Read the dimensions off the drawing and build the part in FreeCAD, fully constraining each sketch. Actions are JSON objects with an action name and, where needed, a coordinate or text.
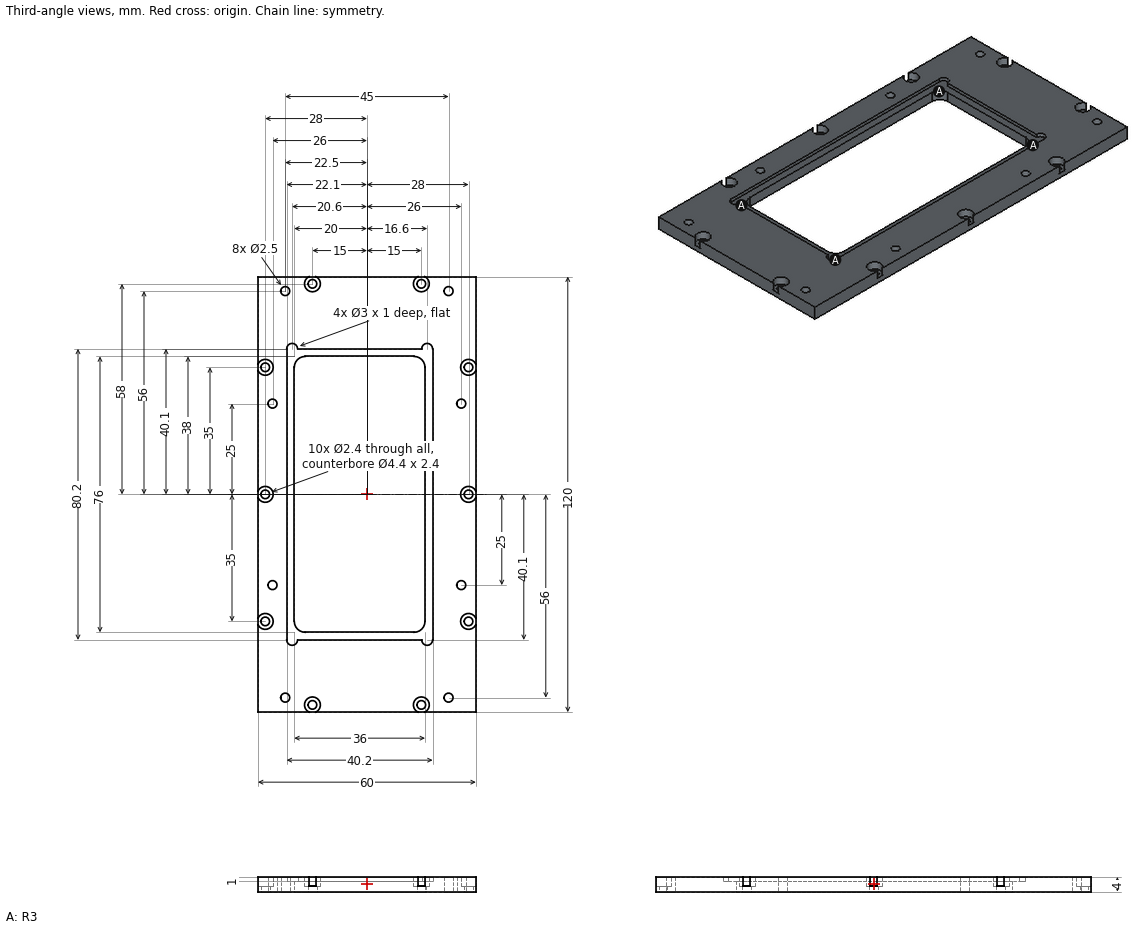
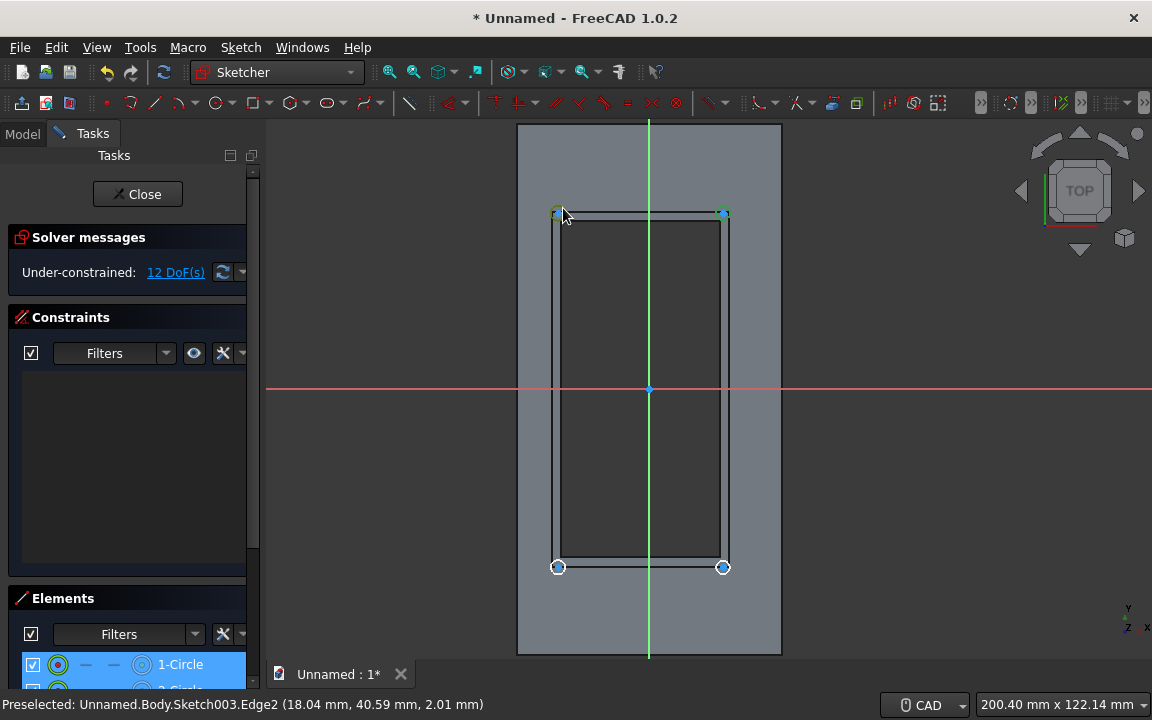
{"action": "scroll", "coordinate": [728, 563], "scroll_direction": "up", "scroll_amount": 4}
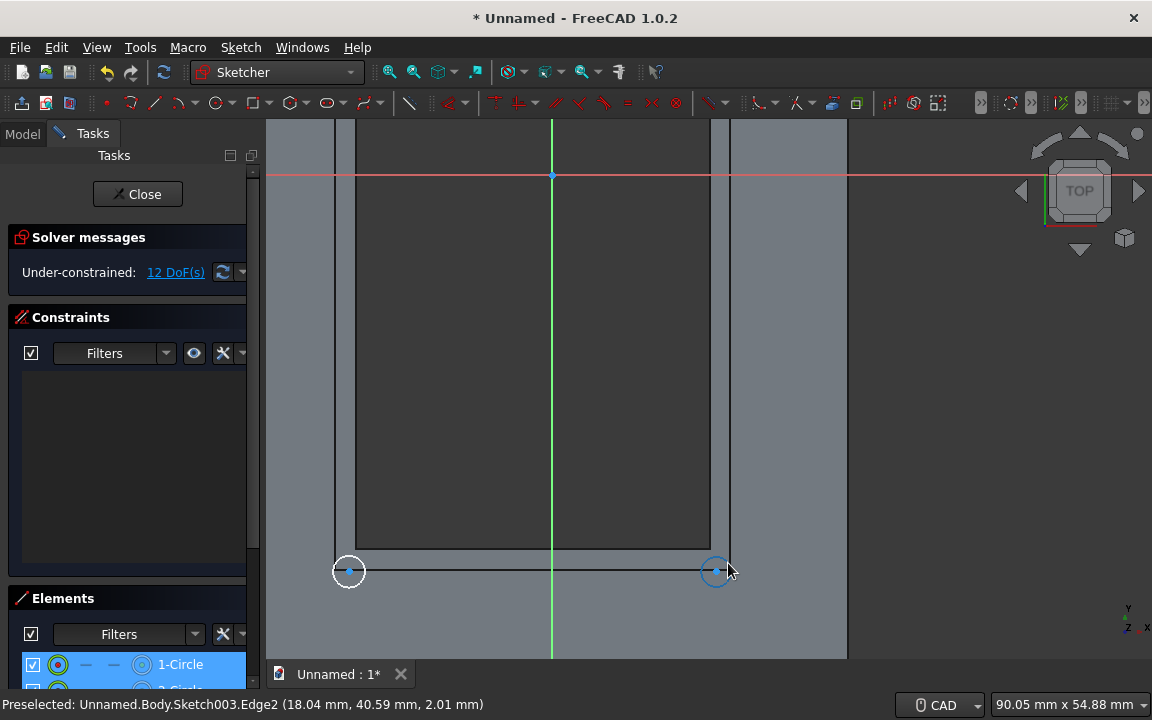
{"action": "left_click", "coordinate": [727, 561]}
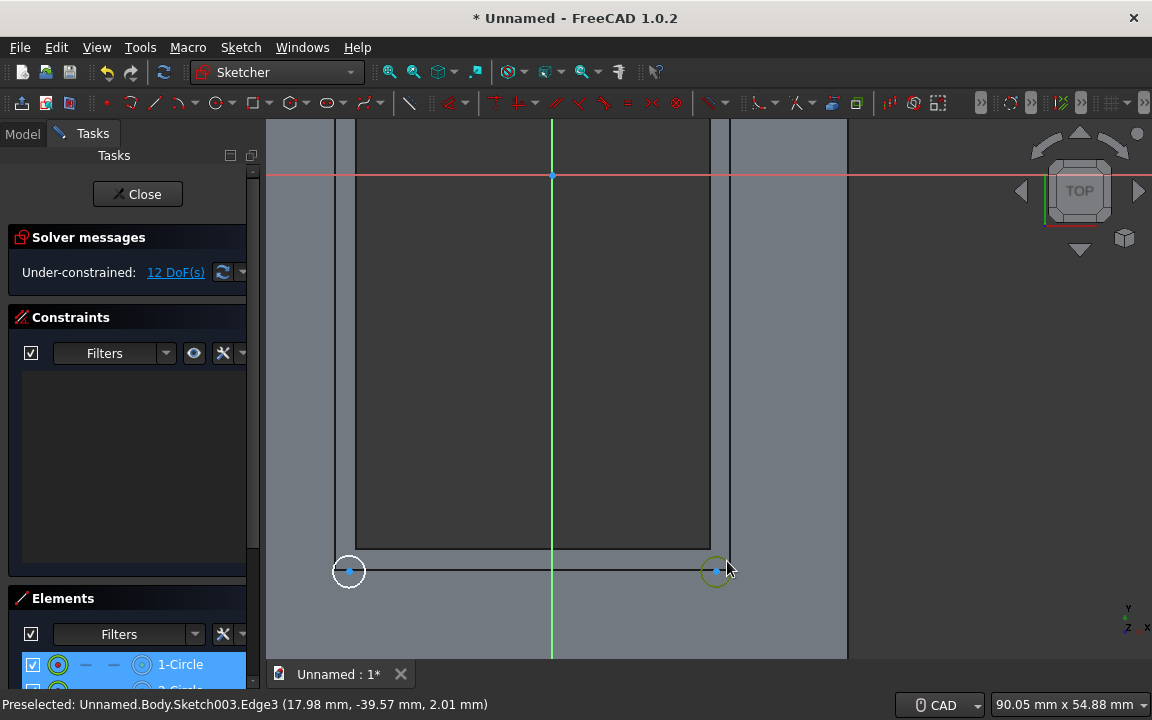
{"action": "left_click", "coordinate": [360, 560]}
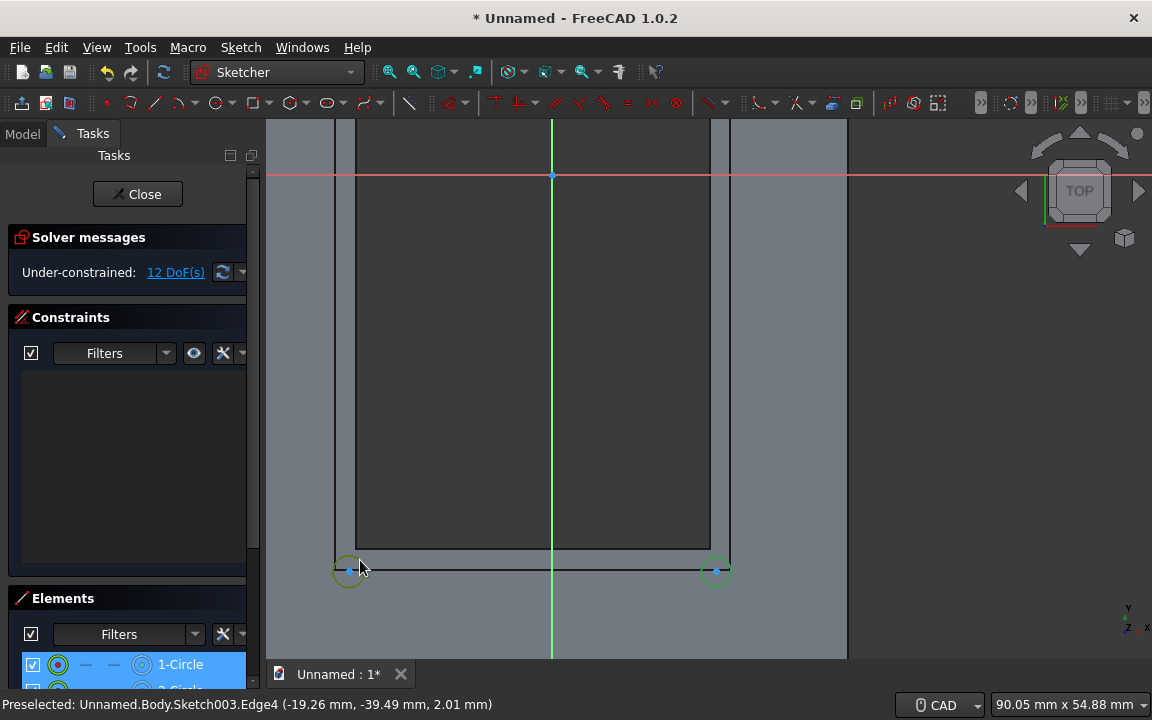
{"action": "key", "text": "e"}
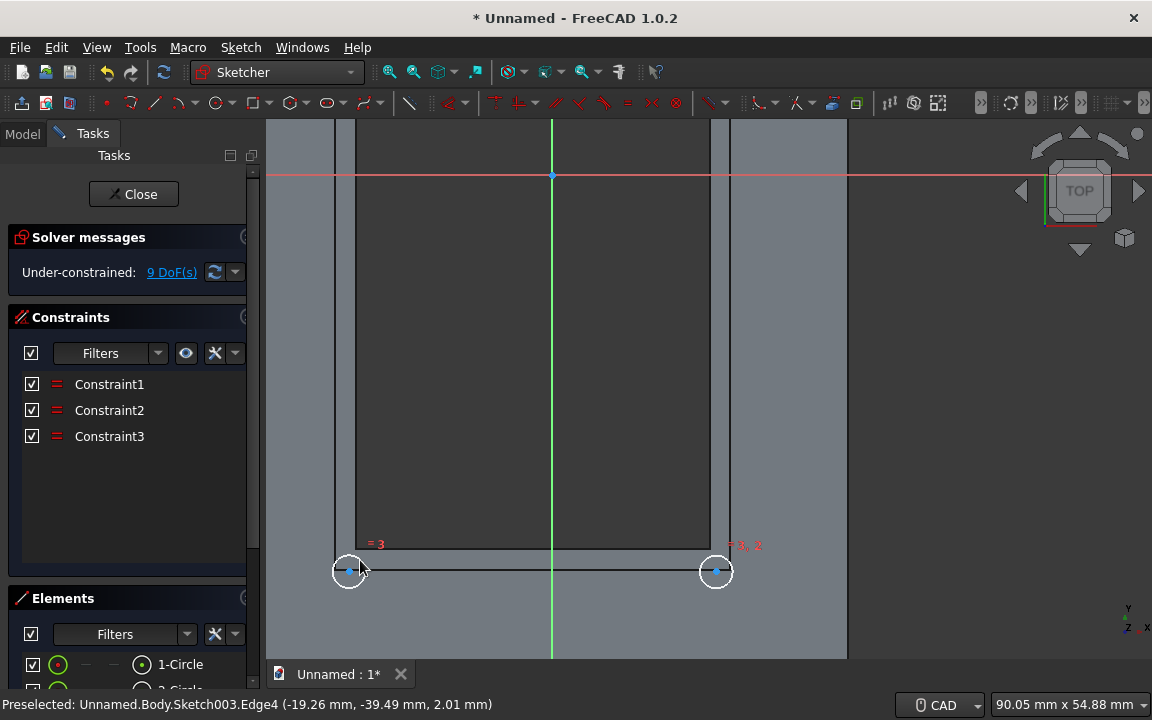
{"action": "scroll", "coordinate": [728, 563], "scroll_direction": "down", "scroll_amount": 4}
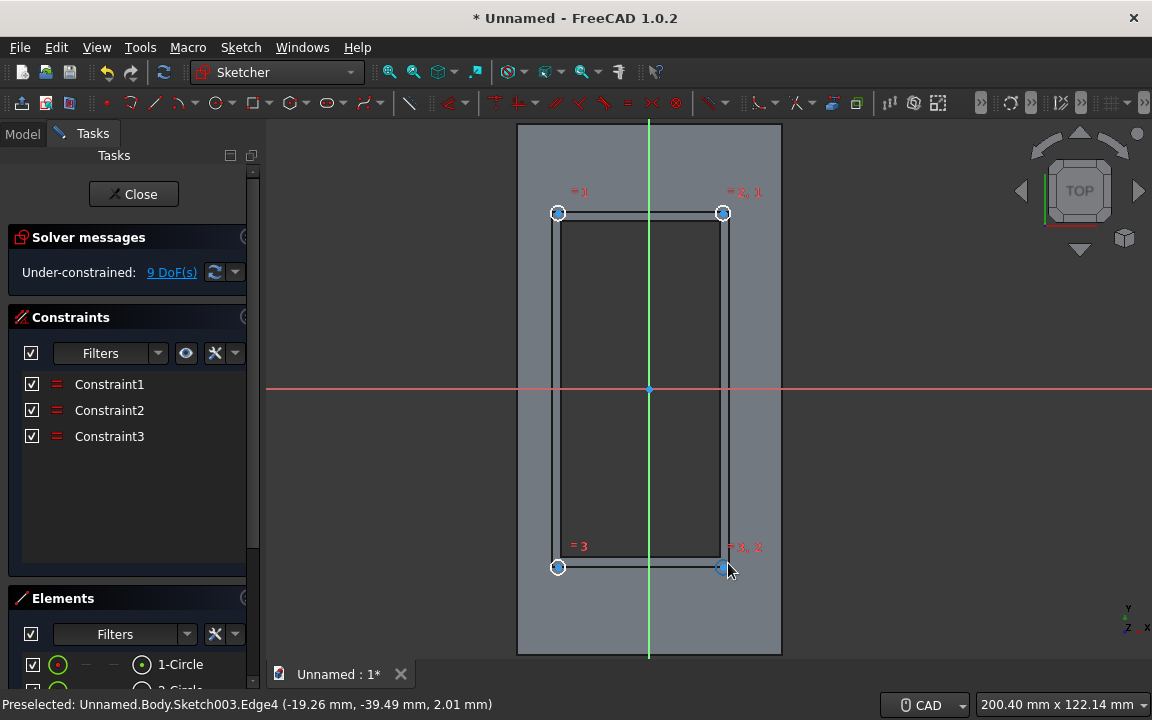
{"action": "left_click", "coordinate": [558, 213]}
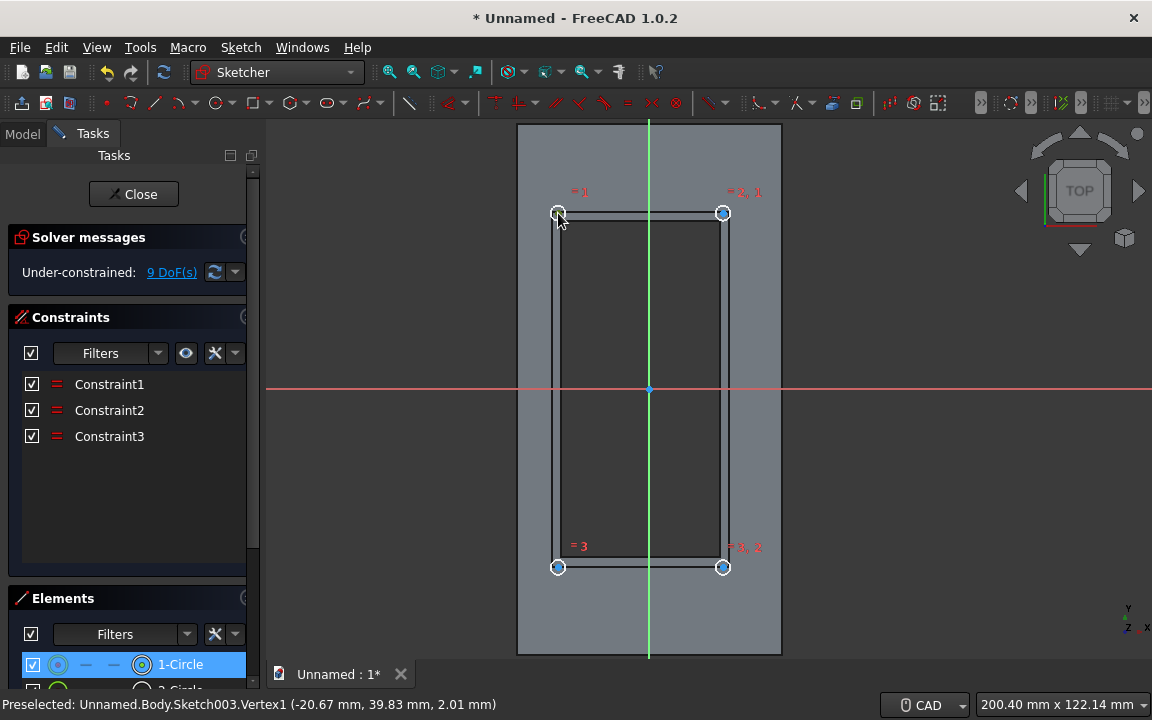
{"action": "left_click", "coordinate": [723, 213]}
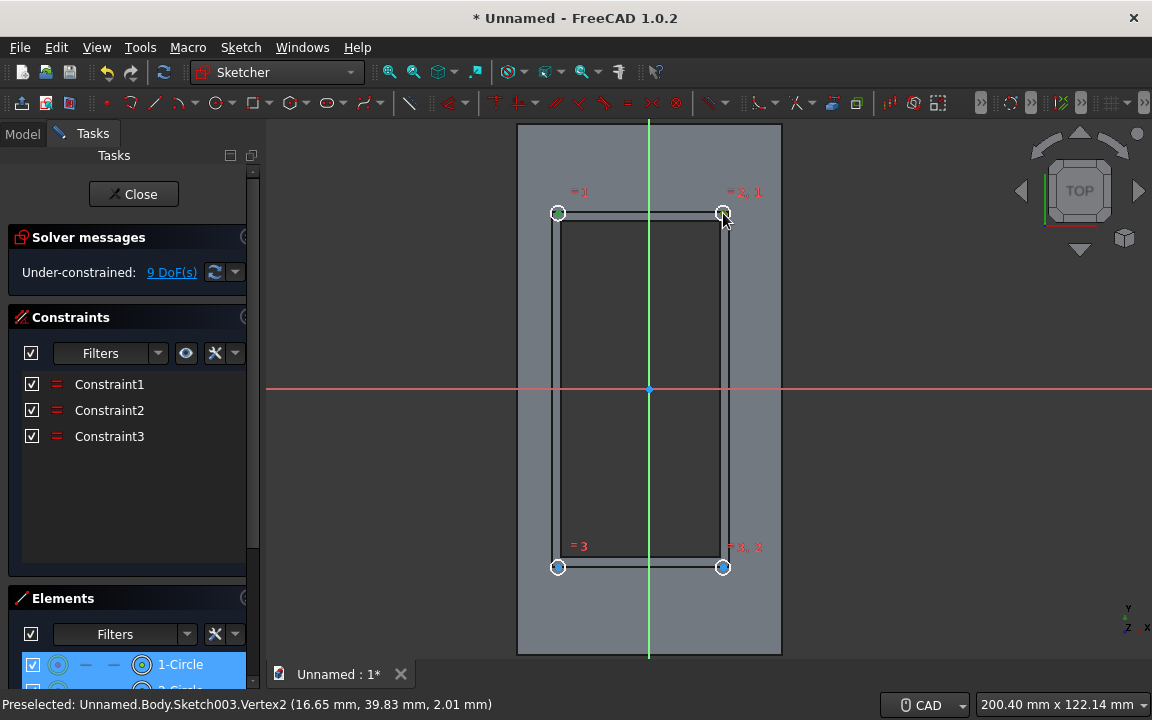
{"action": "key", "text": "h"}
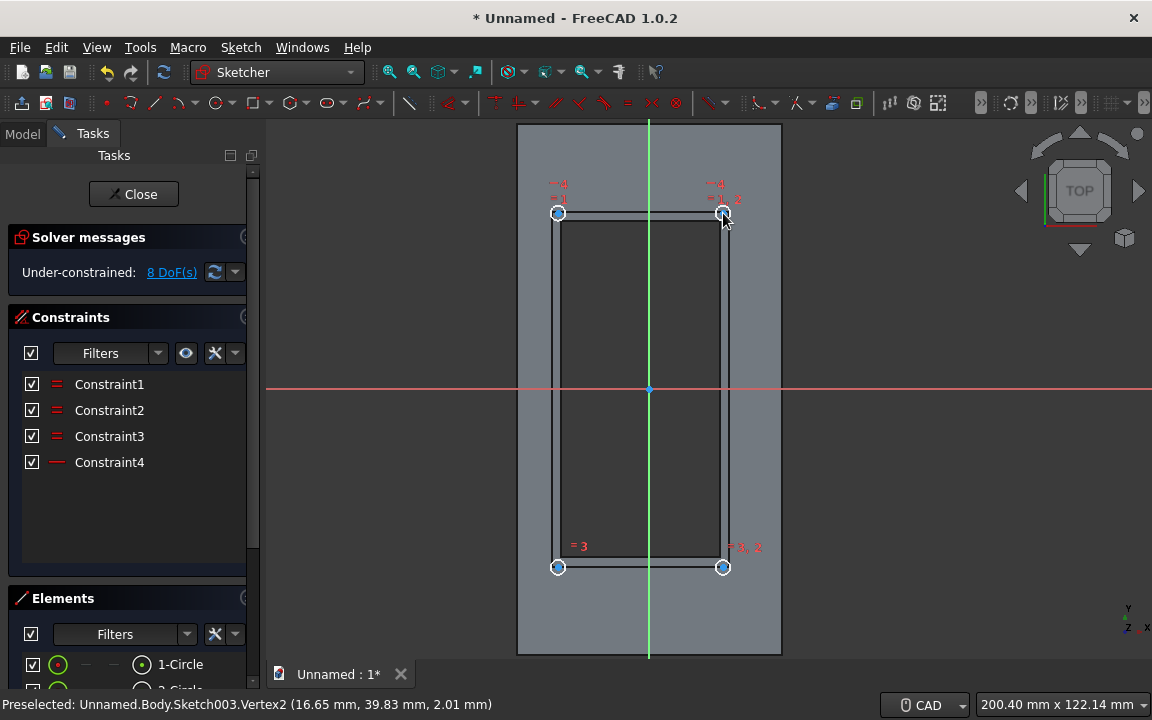
{"action": "left_click", "coordinate": [723, 213]}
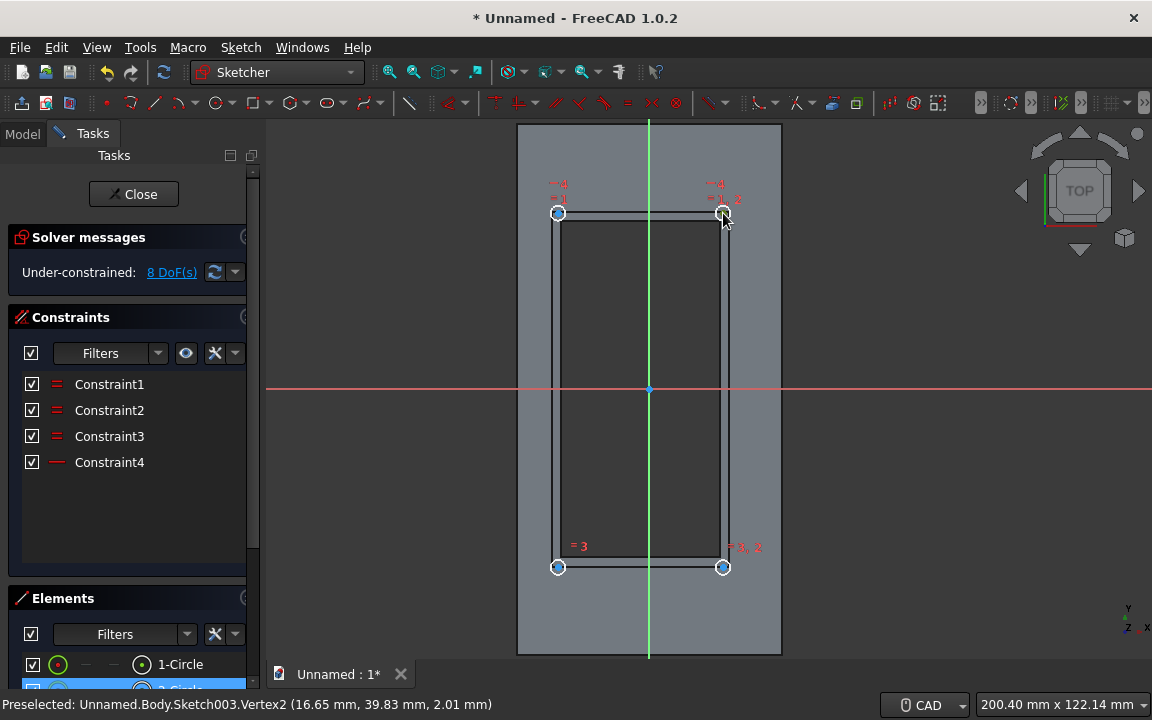
{"action": "left_click", "coordinate": [723, 567]}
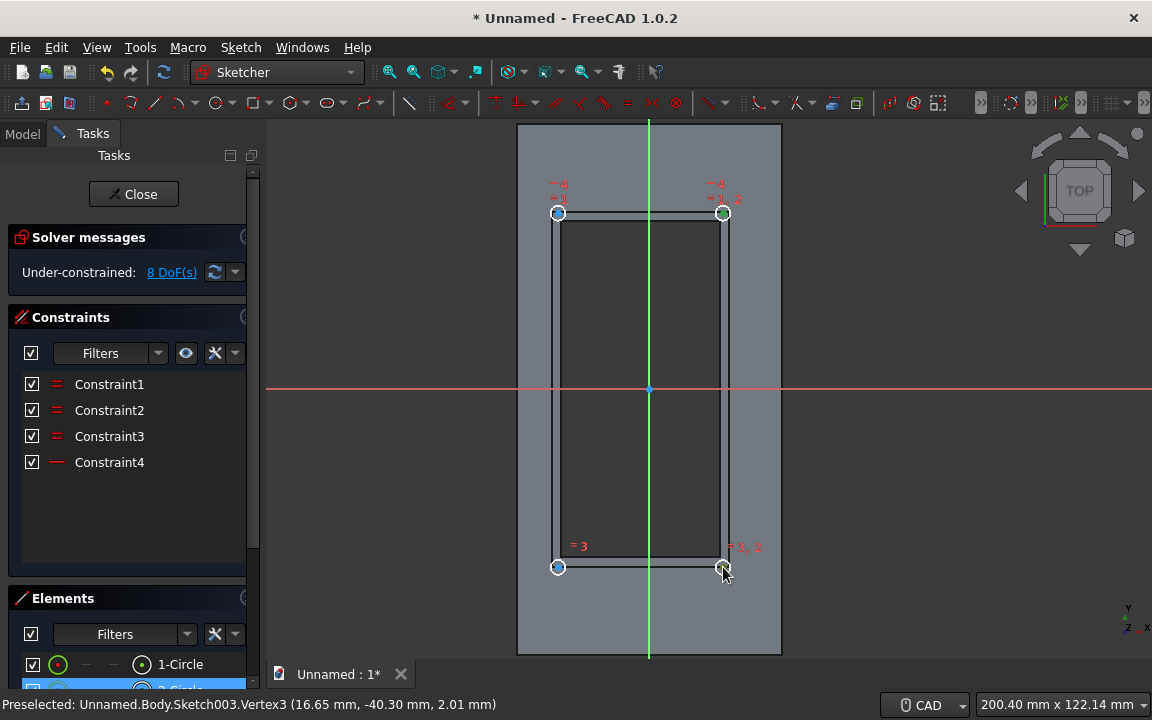
{"action": "left_click", "coordinate": [538, 104]}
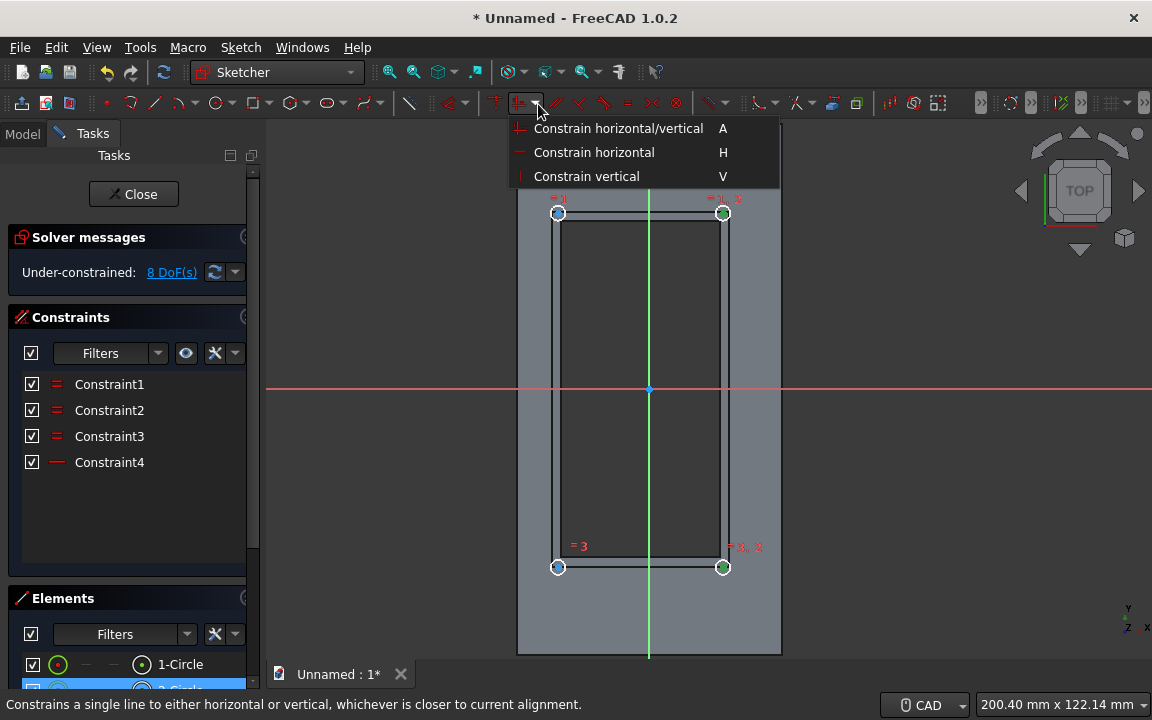
{"action": "left_click", "coordinate": [644, 176]}